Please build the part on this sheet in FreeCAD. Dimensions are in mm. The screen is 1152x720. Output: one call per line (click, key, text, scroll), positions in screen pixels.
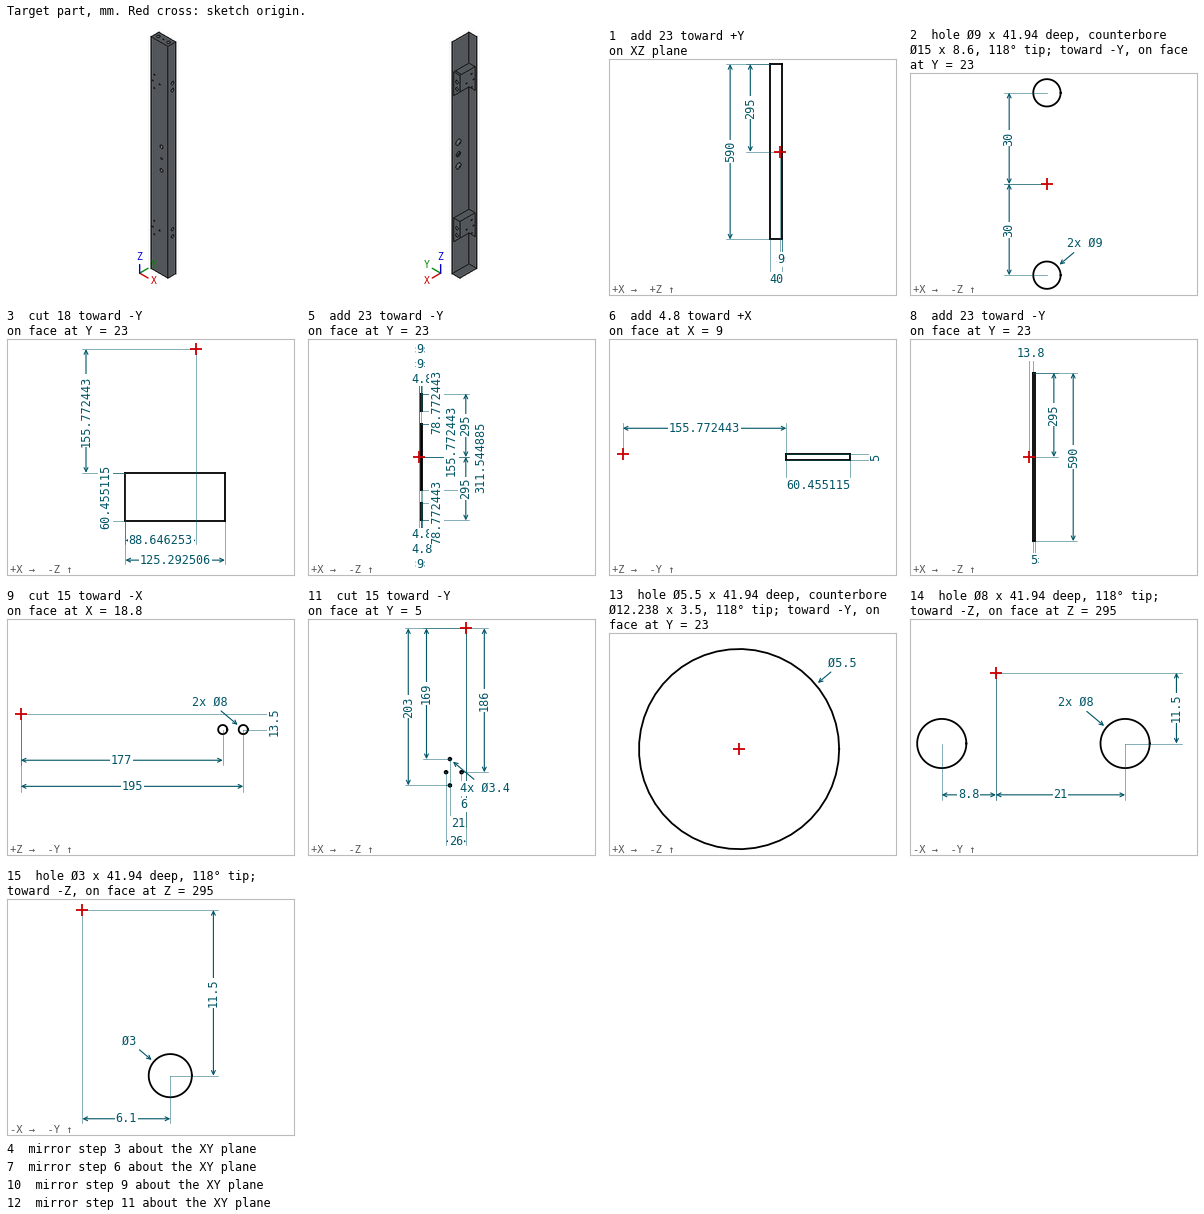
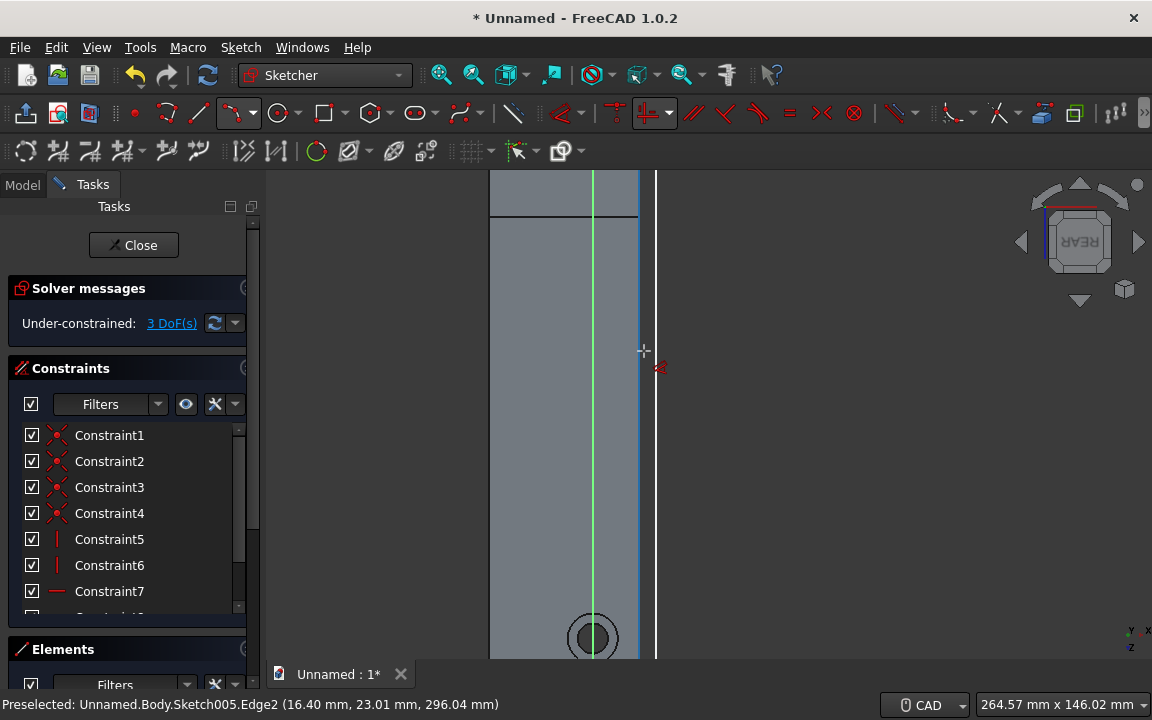
click(639, 346)
click(673, 414)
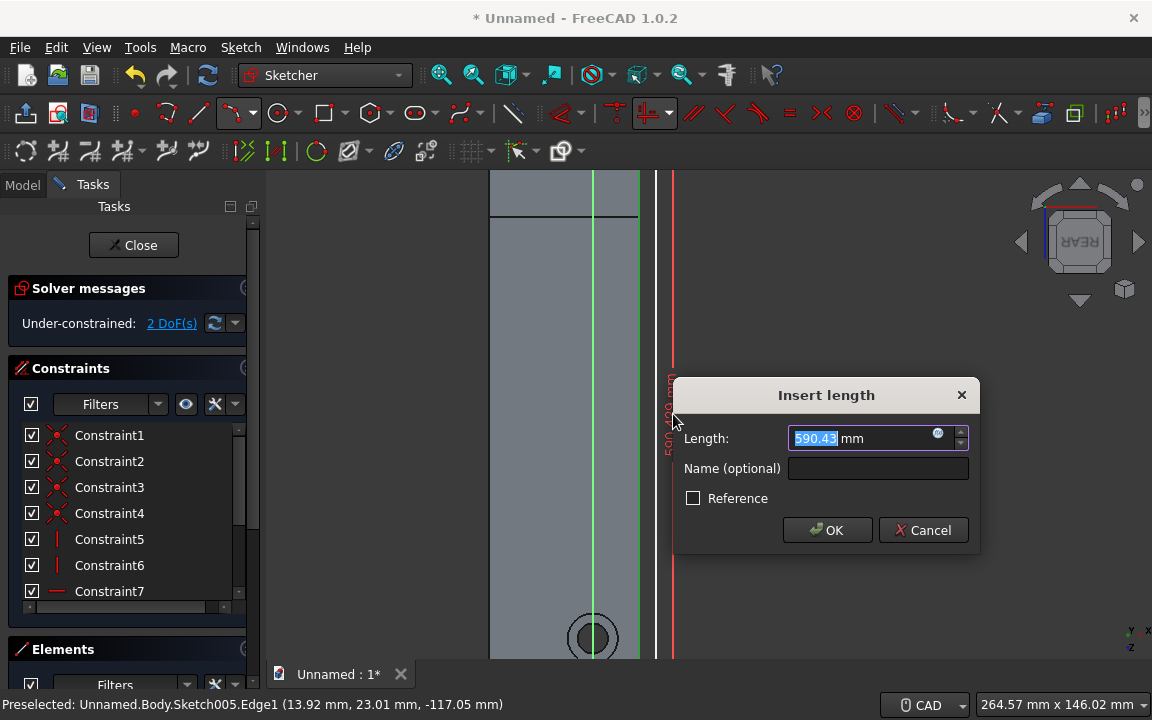
text(590)
key(Return)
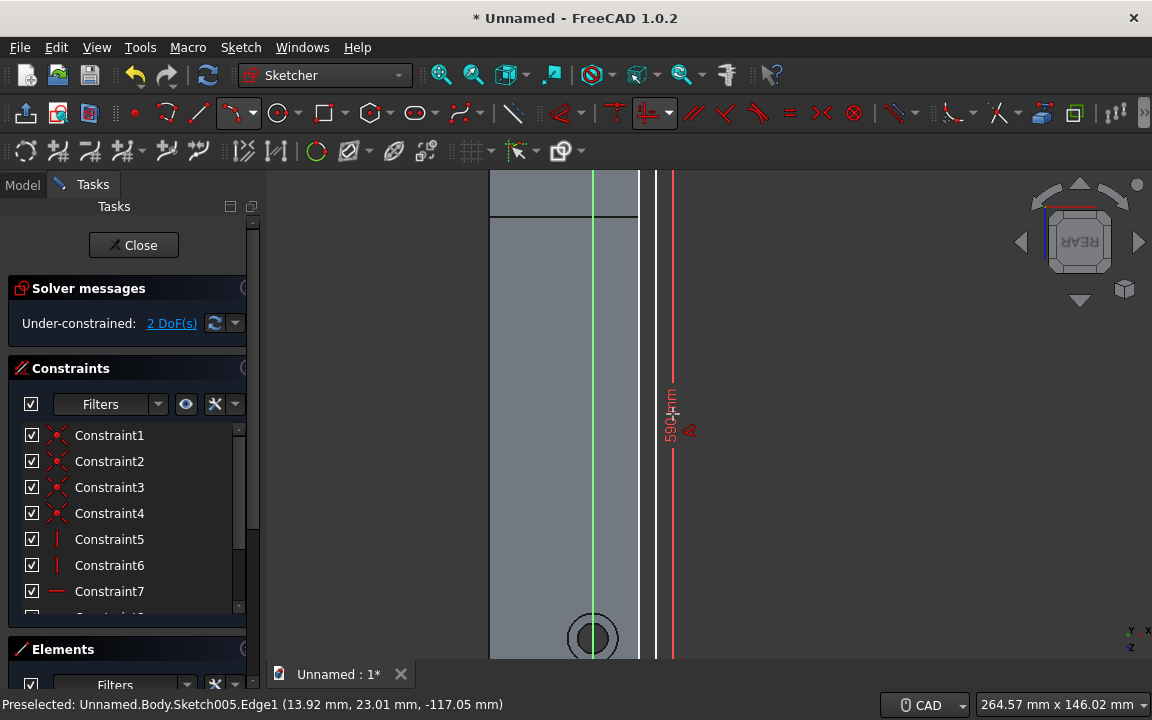
scroll(644, 350, down, 9)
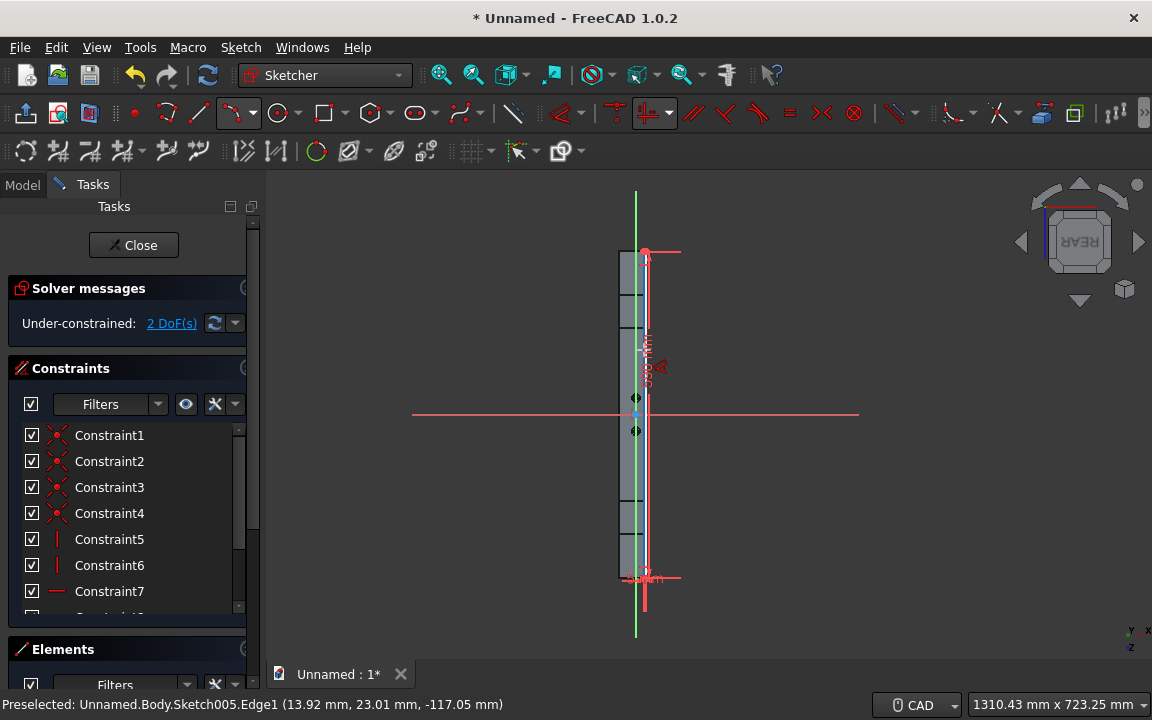
scroll(644, 252, up, 8)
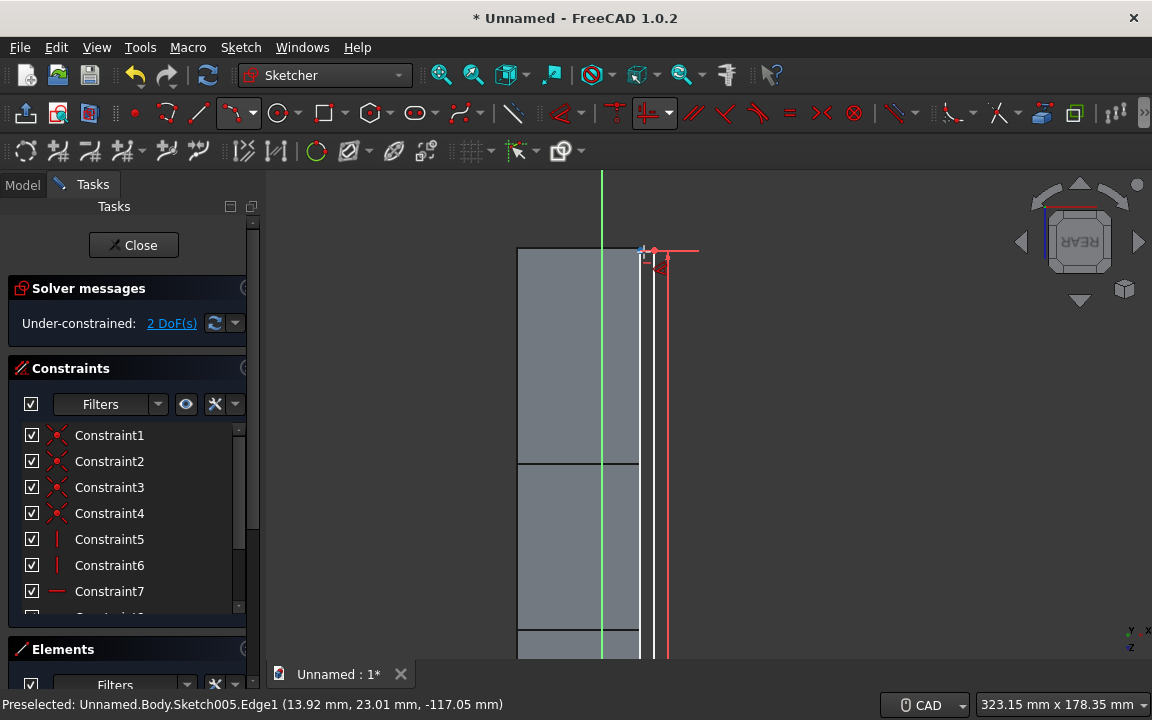
click(640, 251)
click(568, 441)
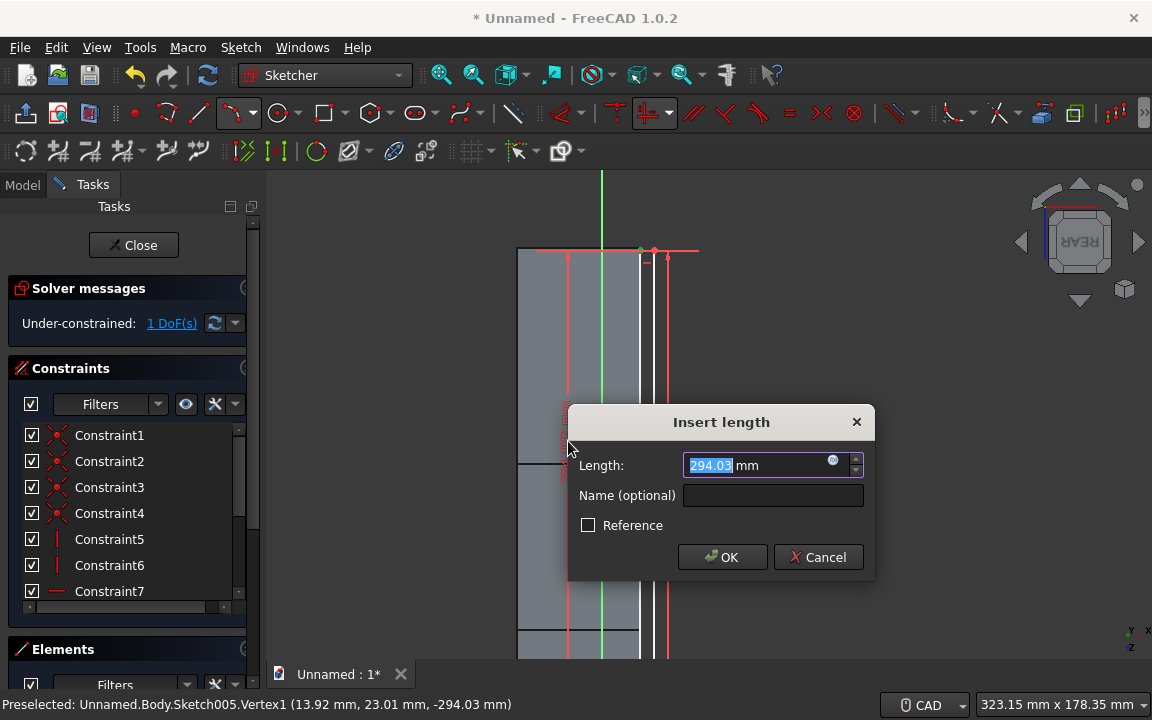
text(295)
key(Return)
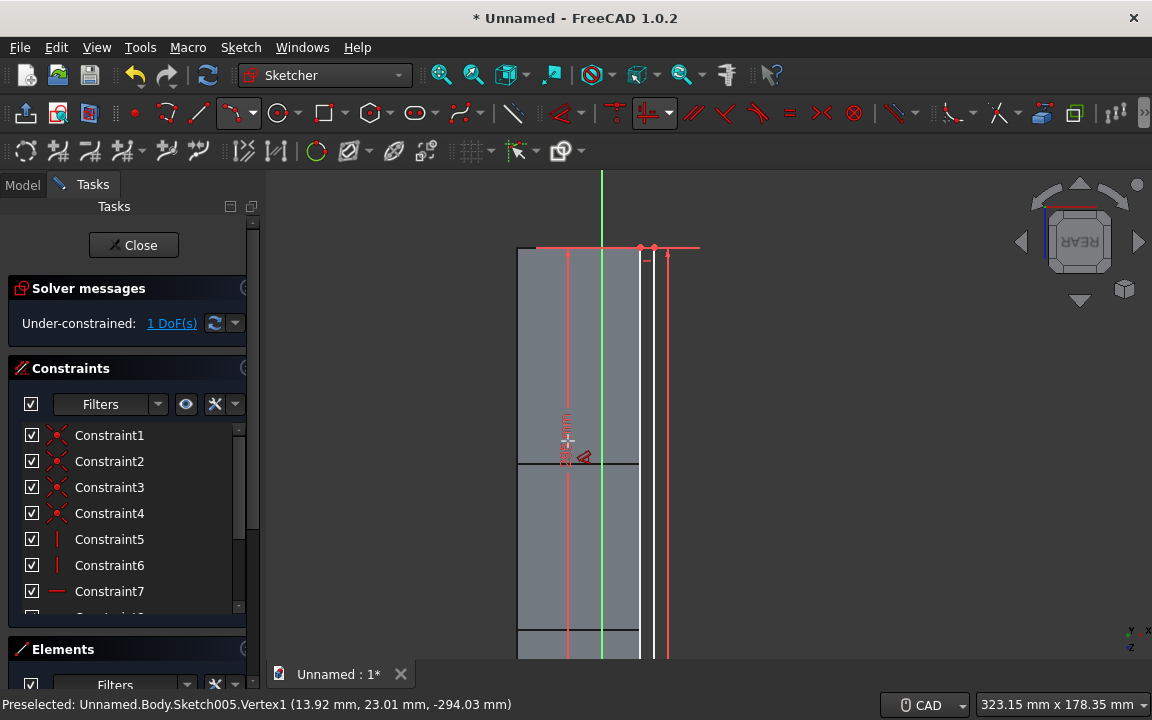
click(640, 248)
click(621, 214)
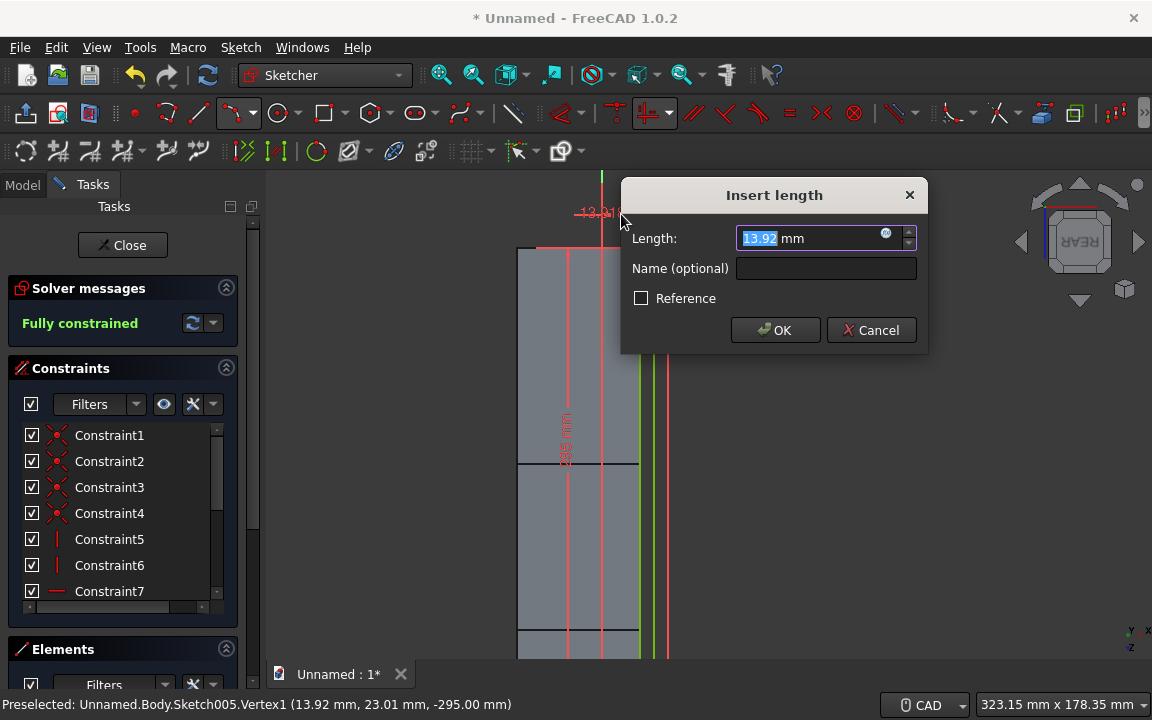
text(13.8)
key(Return)
key(Escape)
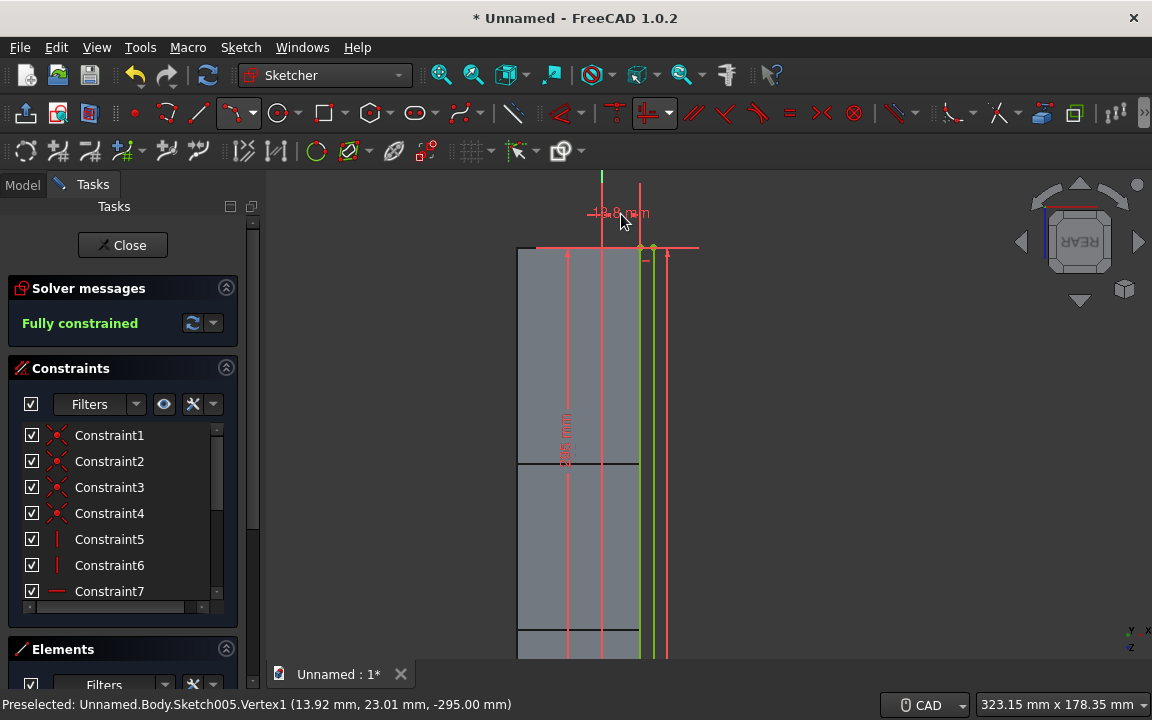
click(123, 245)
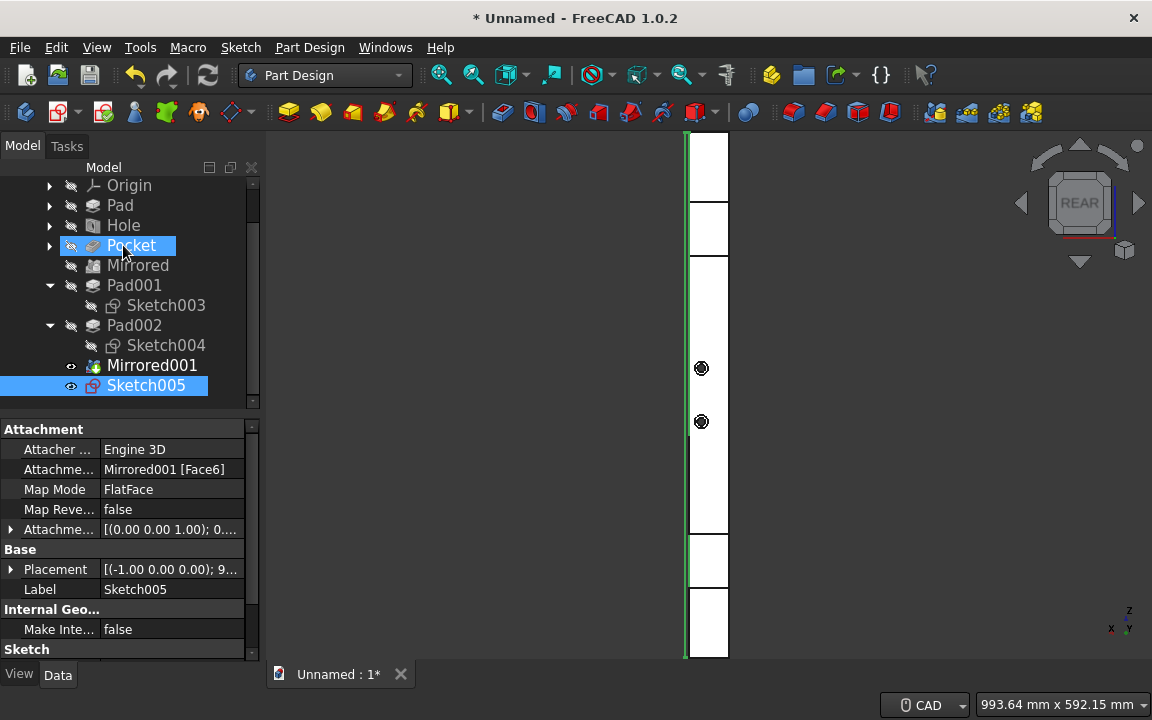
click(290, 112)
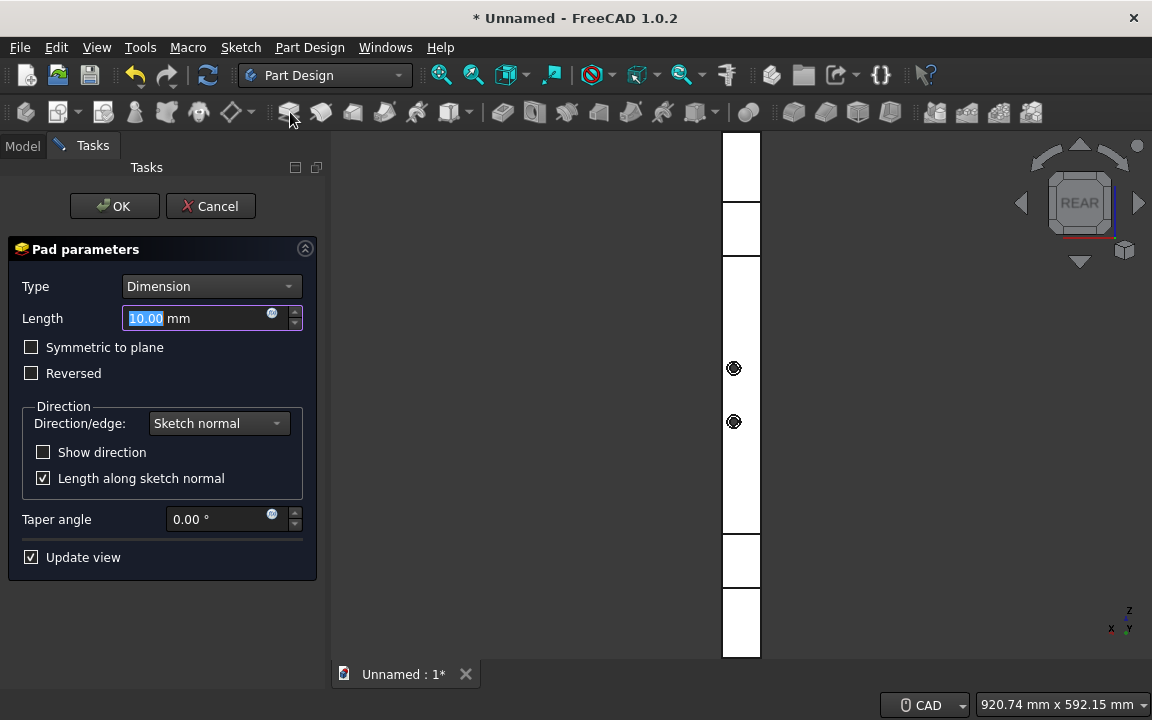
text(23)
key(Tab)